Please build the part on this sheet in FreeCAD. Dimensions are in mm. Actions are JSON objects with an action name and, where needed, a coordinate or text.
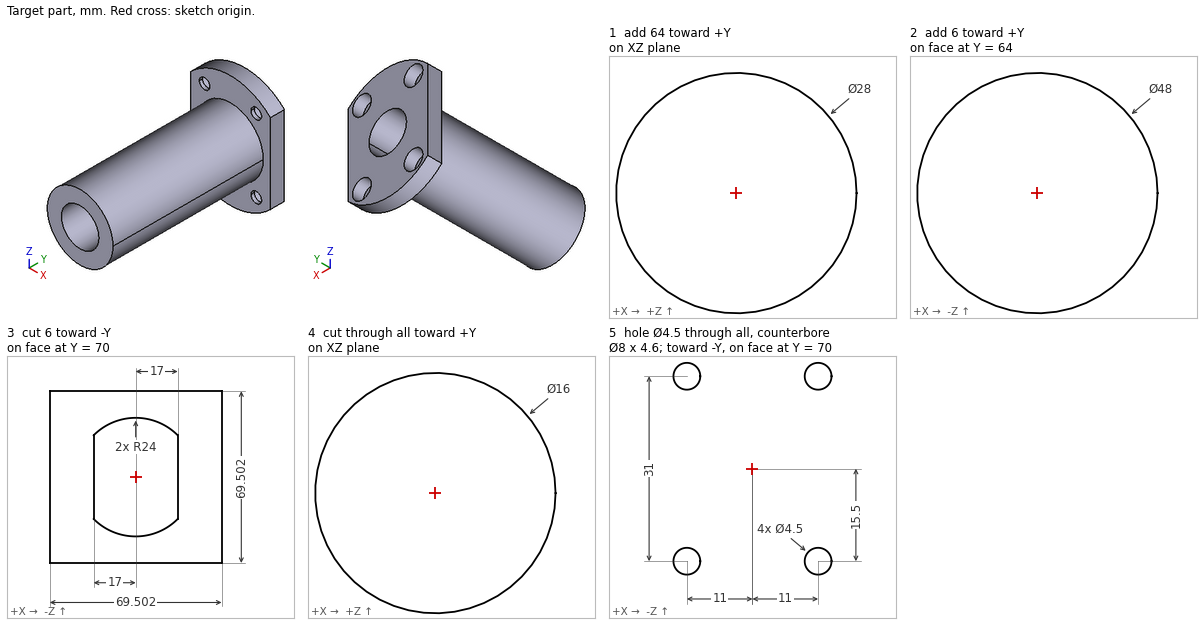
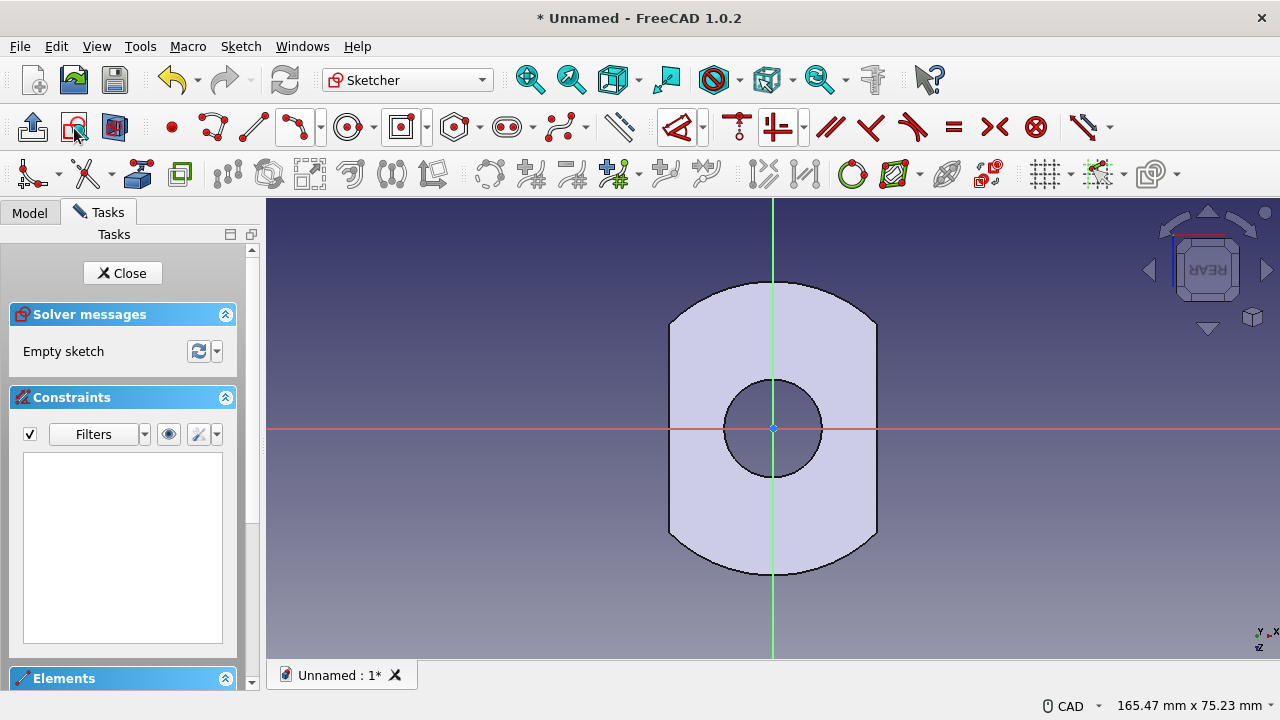
{"action": "key", "text": "g c"}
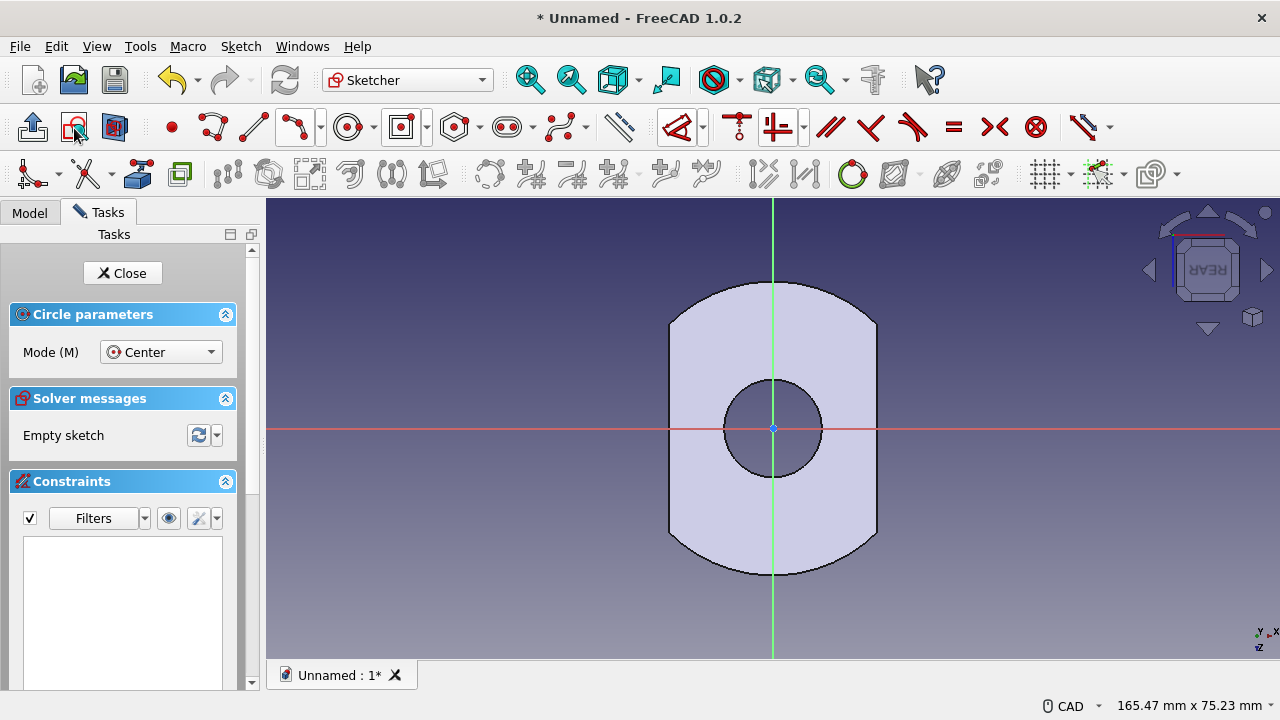
{"action": "scroll", "coordinate": [840, 523], "scroll_direction": "up", "scroll_amount": 3}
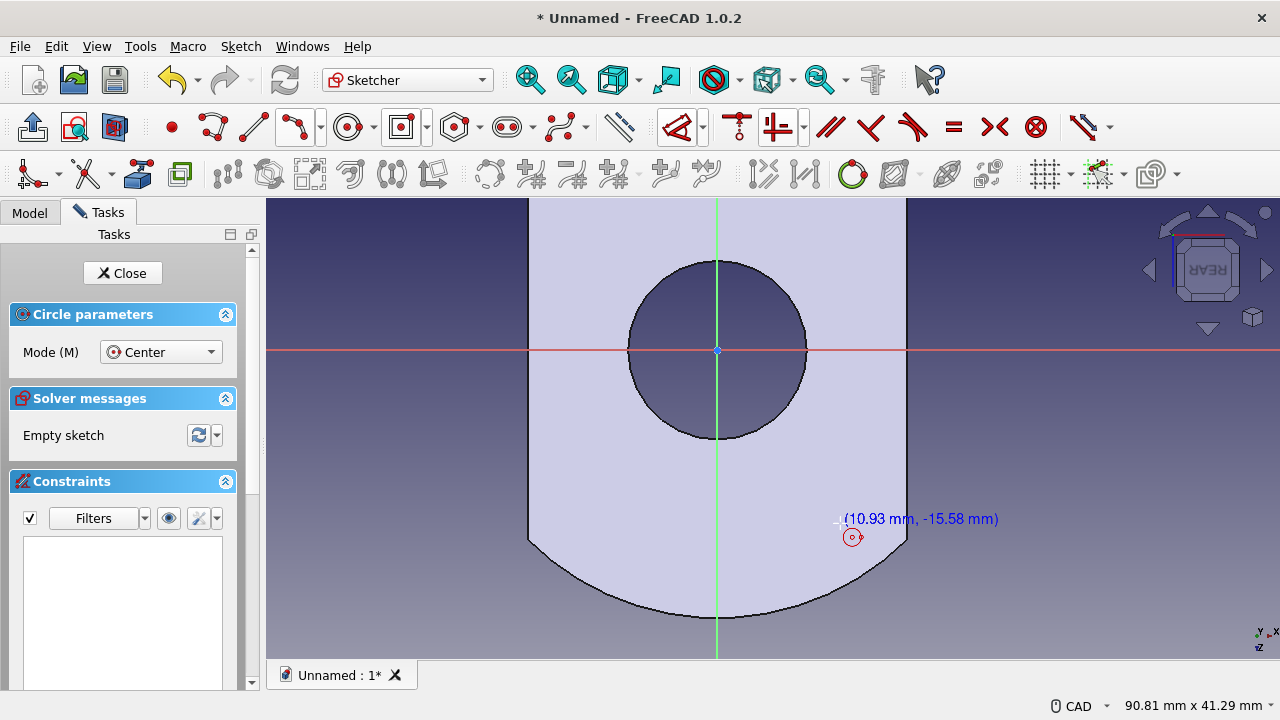
{"action": "left_click", "coordinate": [840, 523]}
{"action": "left_click", "coordinate": [858, 506]}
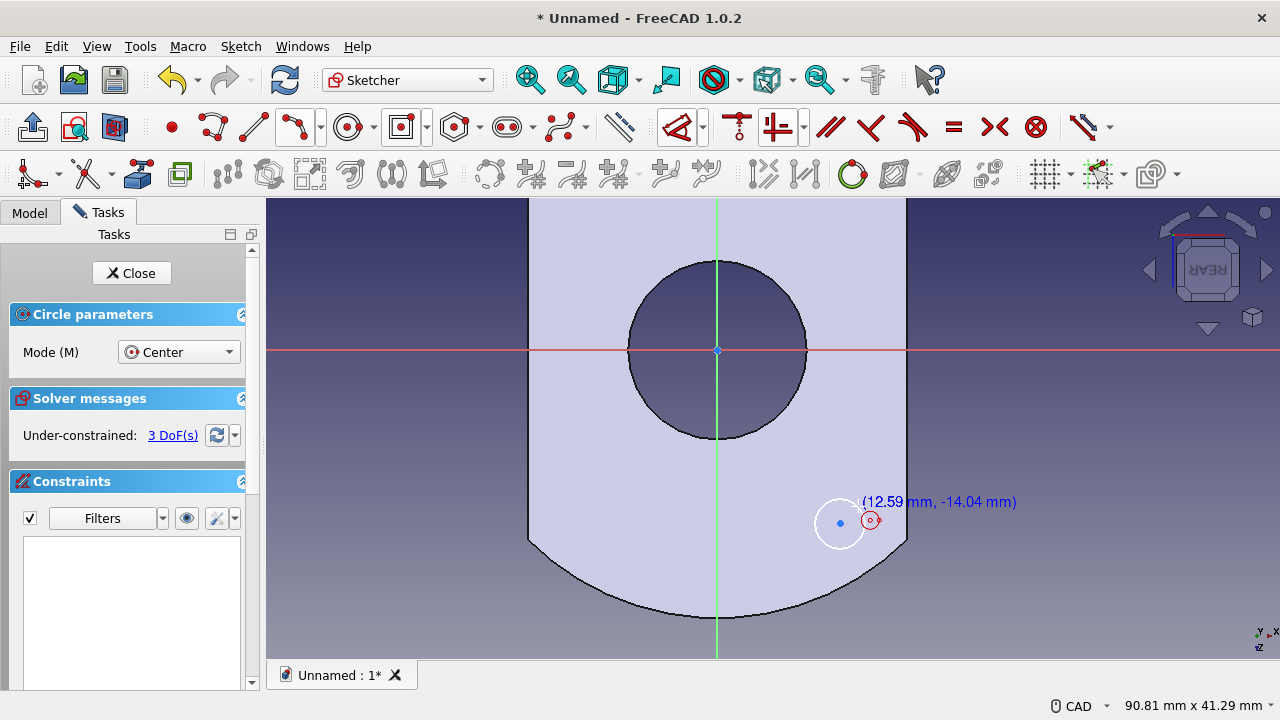
{"action": "left_click", "coordinate": [595, 523]}
{"action": "left_click", "coordinate": [612, 506]}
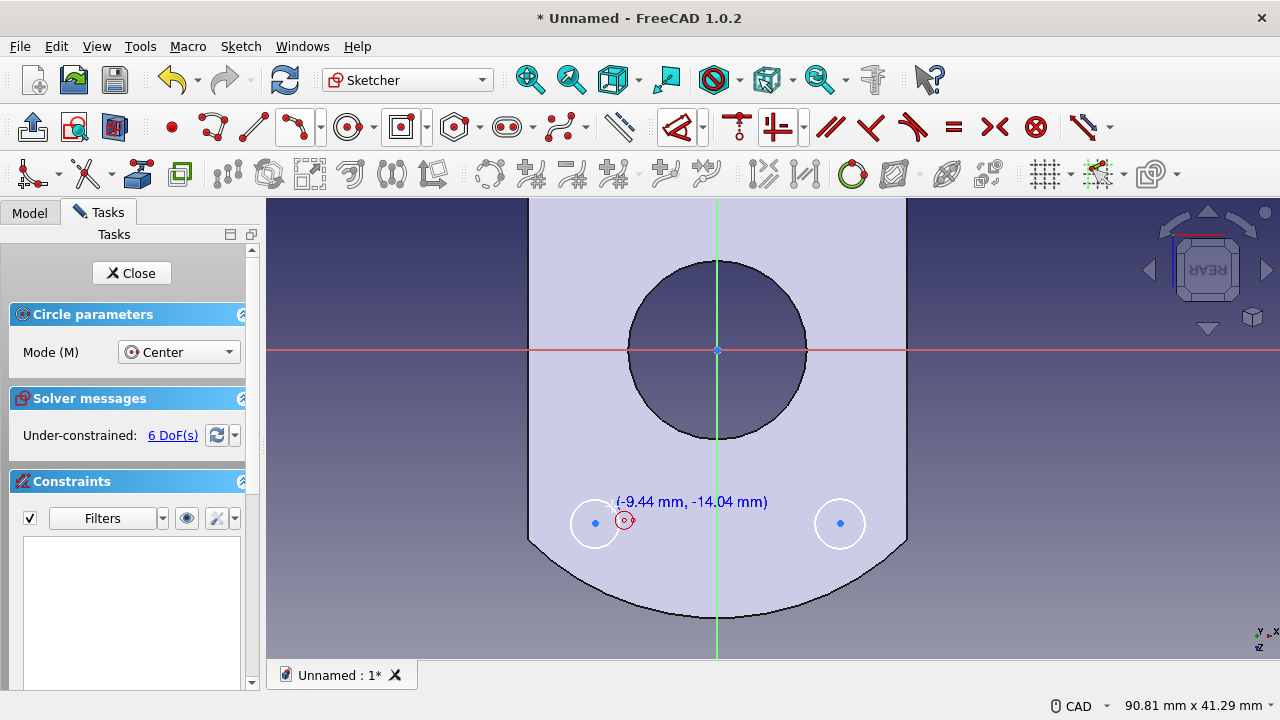
{"action": "scroll", "coordinate": [678, 588], "scroll_direction": "down", "scroll_amount": 2}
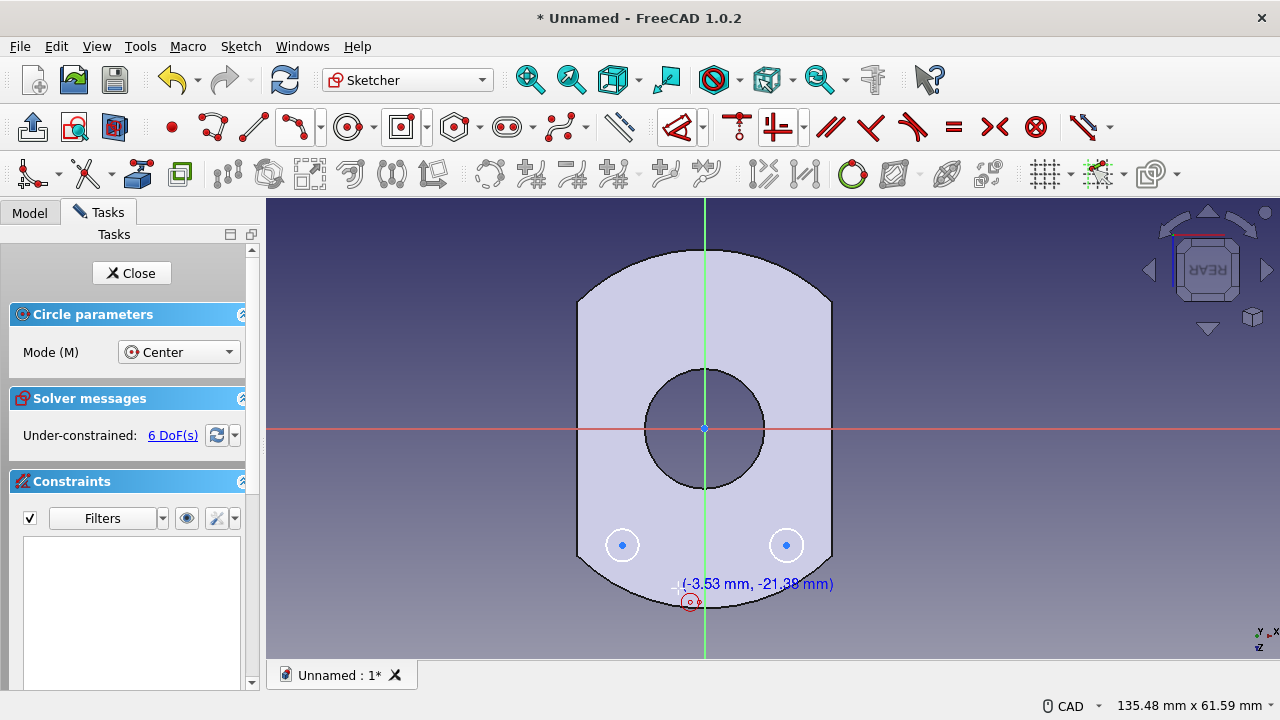
{"action": "scroll", "coordinate": [622, 313], "scroll_direction": "up", "scroll_amount": 2}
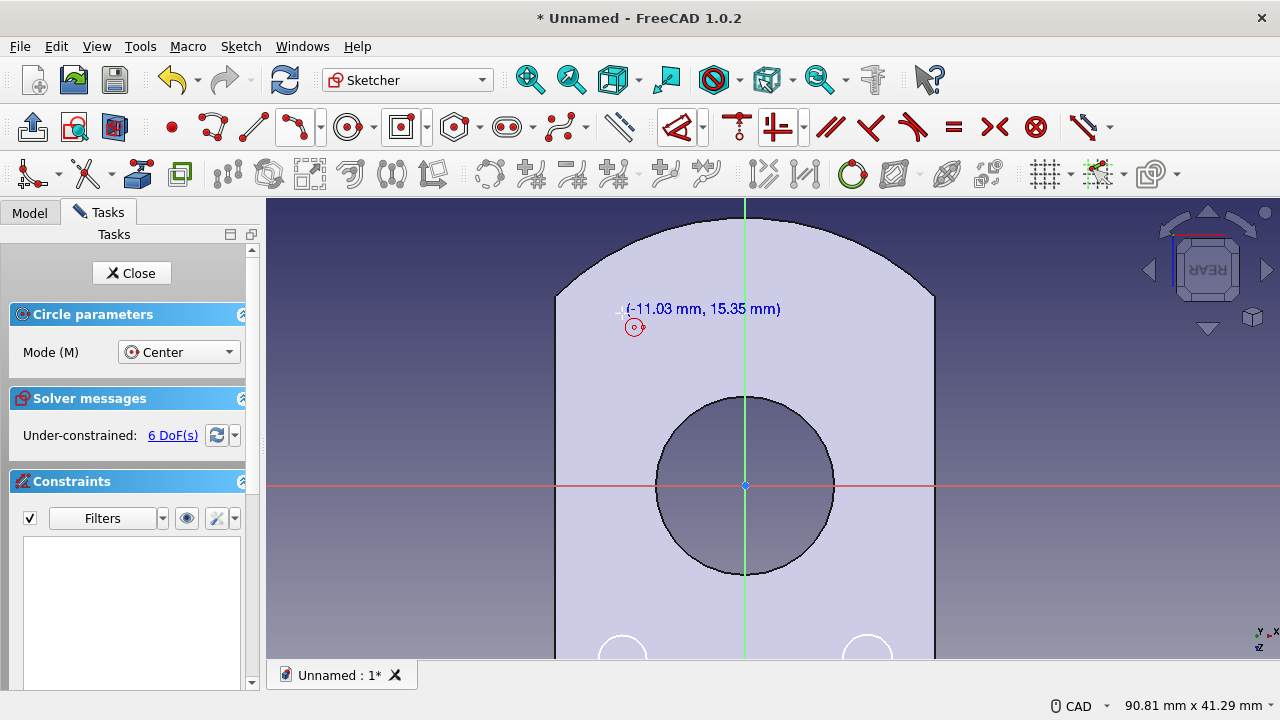
{"action": "left_click", "coordinate": [622, 313]}
{"action": "left_click", "coordinate": [640, 295]}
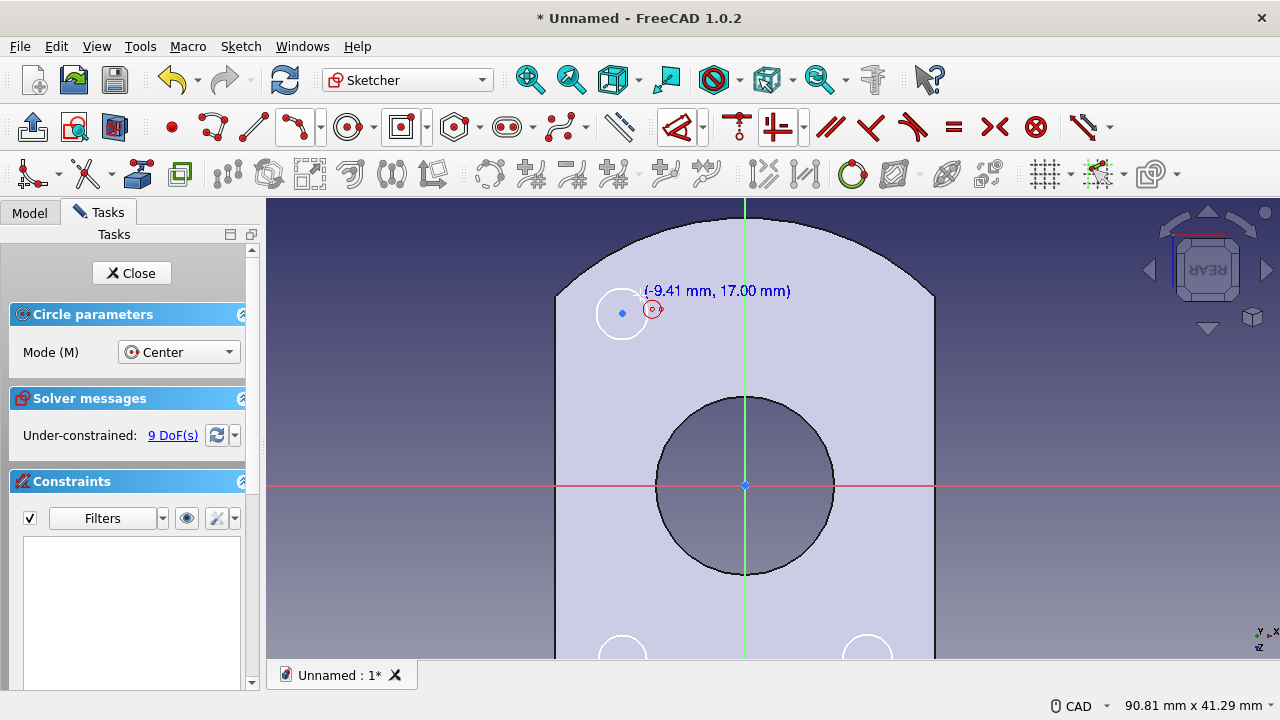
{"action": "left_click", "coordinate": [868, 313]}
{"action": "left_click", "coordinate": [886, 295]}
{"action": "key", "text": "Escape"}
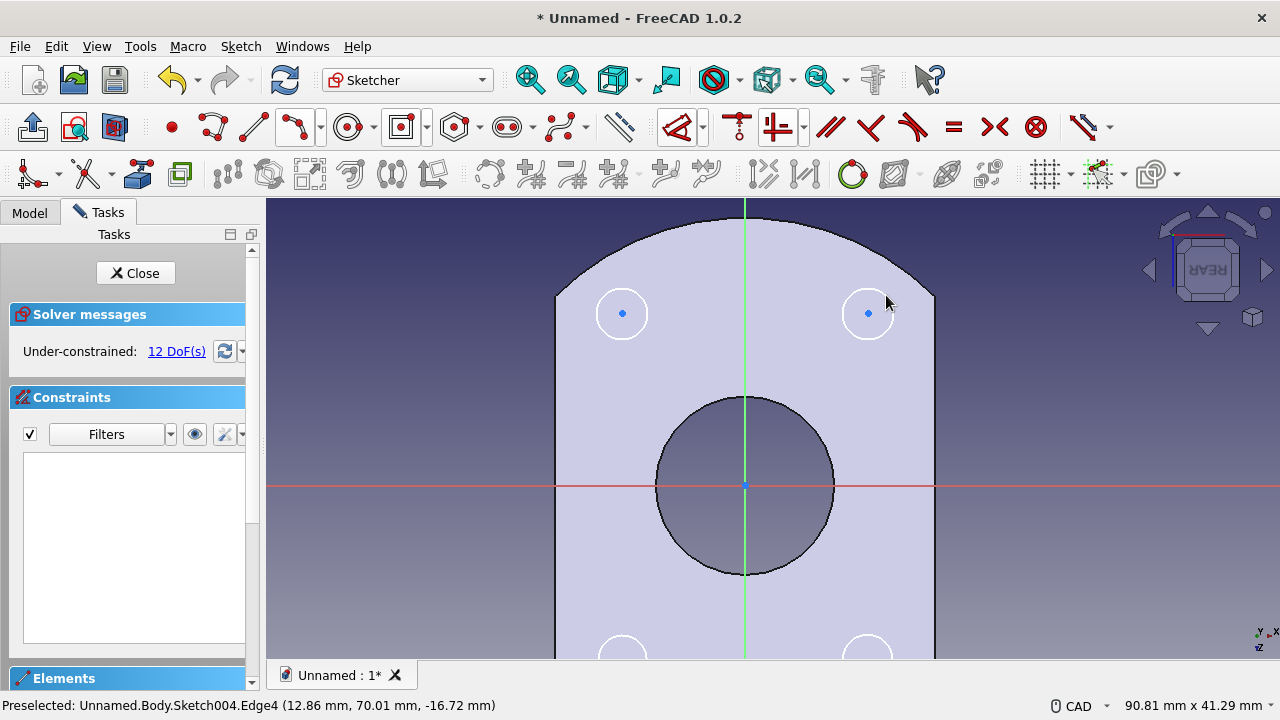
{"action": "scroll", "coordinate": [622, 312], "scroll_direction": "down", "scroll_amount": 2}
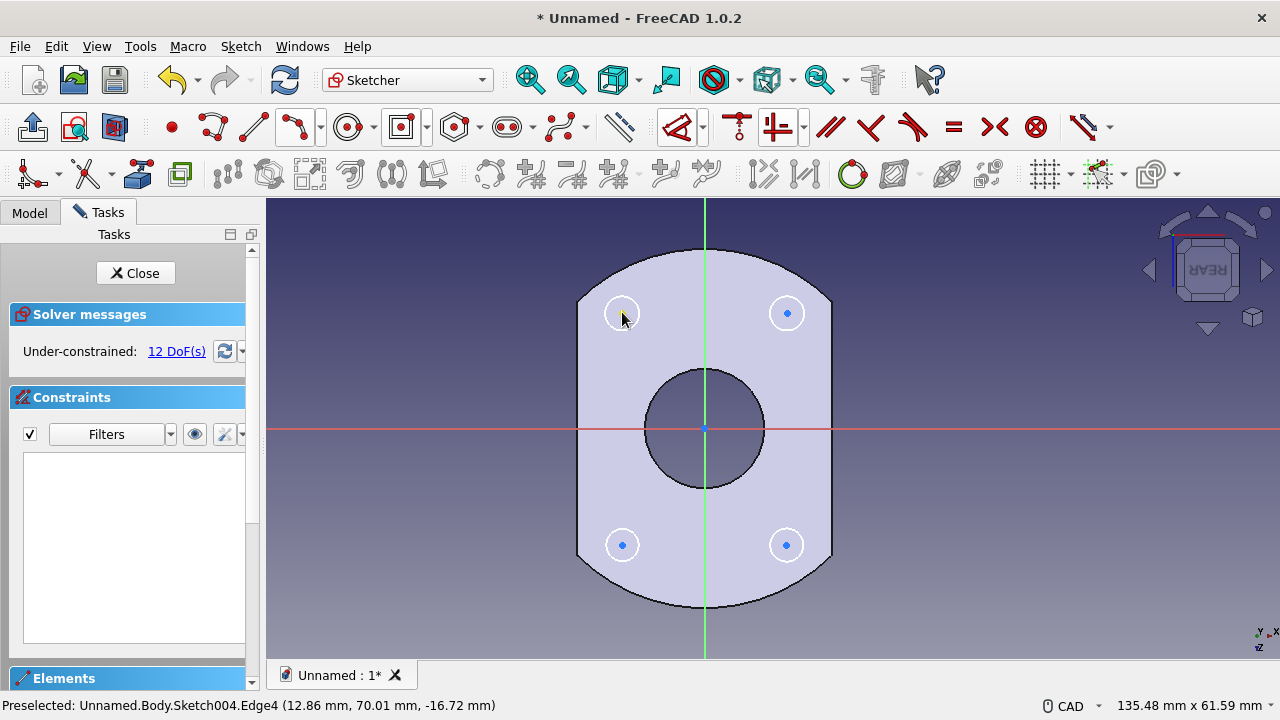
{"action": "left_click", "coordinate": [798, 533]}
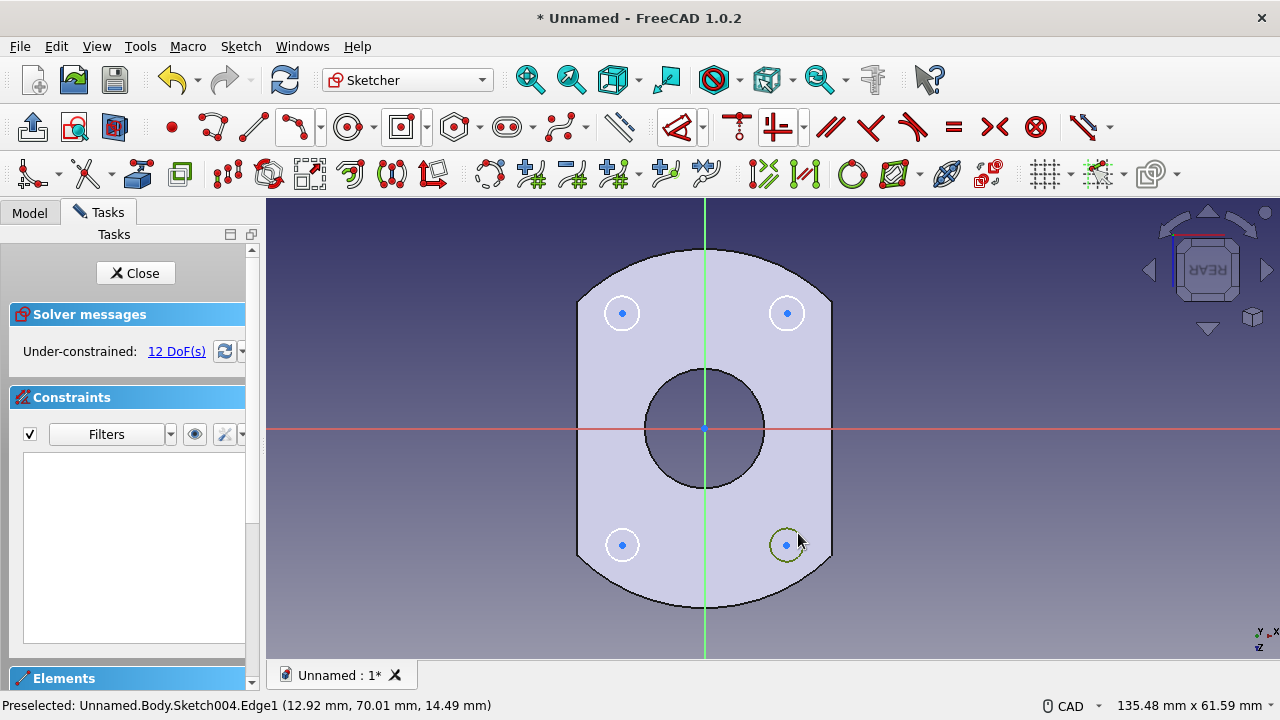
{"action": "left_click", "coordinate": [634, 534]}